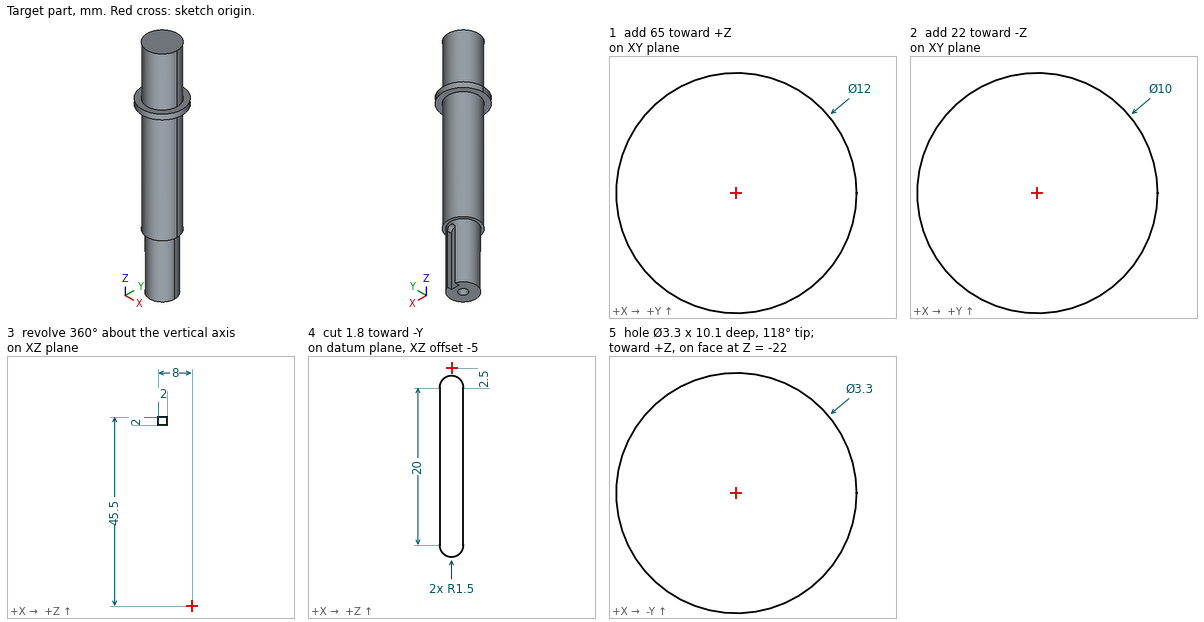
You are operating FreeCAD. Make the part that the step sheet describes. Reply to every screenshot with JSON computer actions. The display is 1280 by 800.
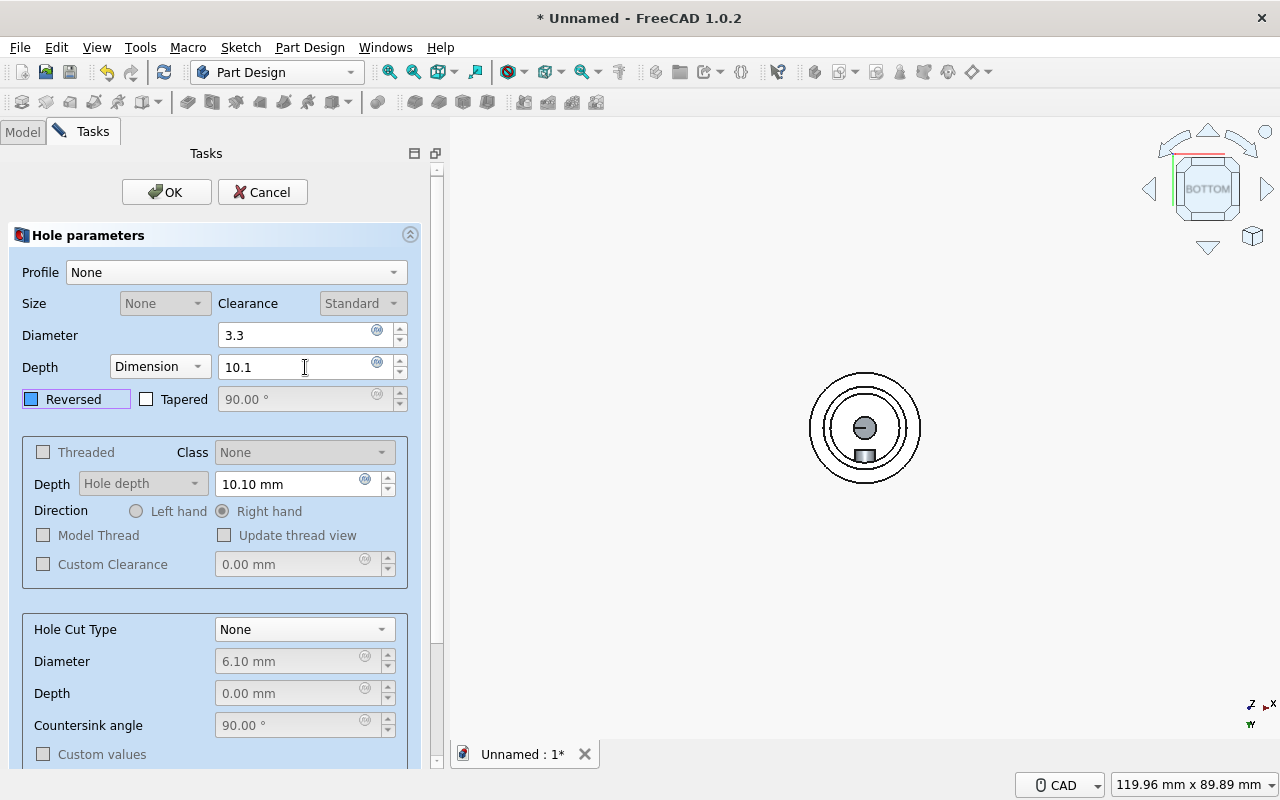
{"action": "left_click", "coordinate": [167, 192]}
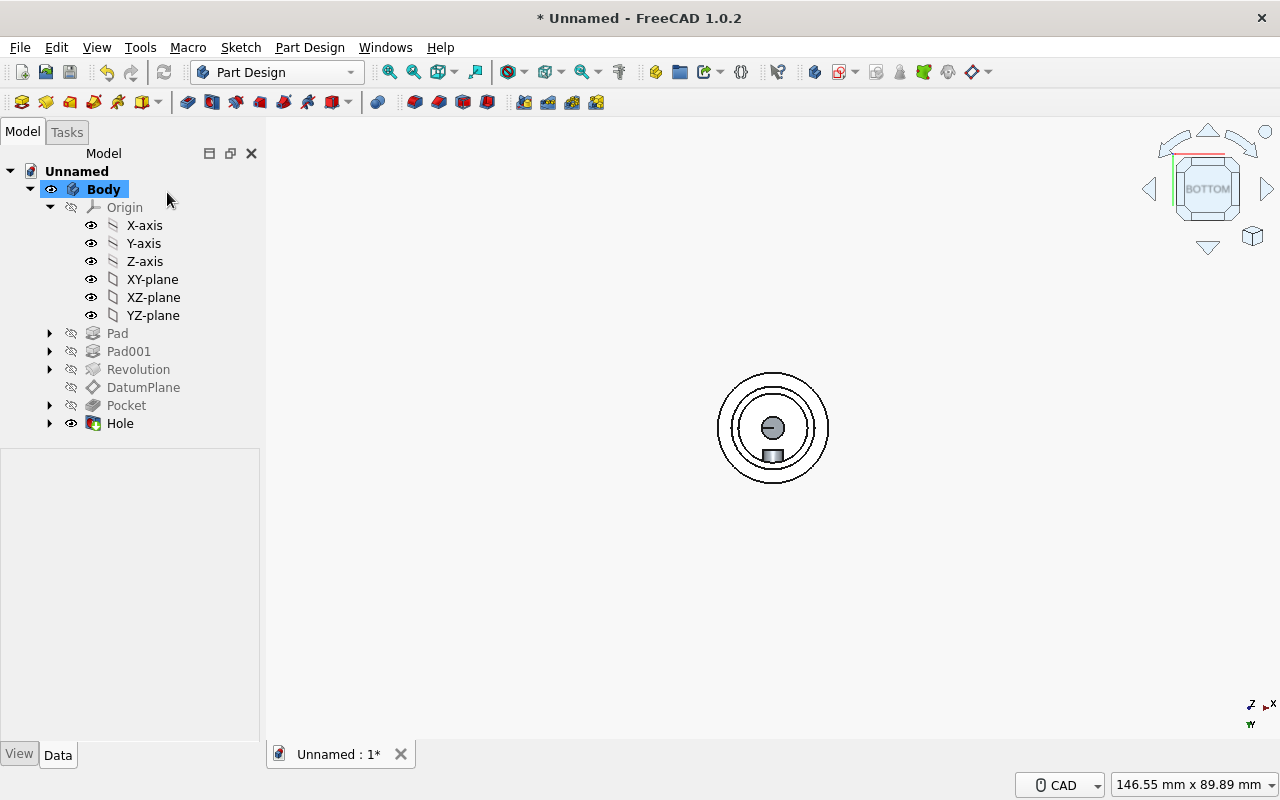
{"action": "key", "text": "0"}